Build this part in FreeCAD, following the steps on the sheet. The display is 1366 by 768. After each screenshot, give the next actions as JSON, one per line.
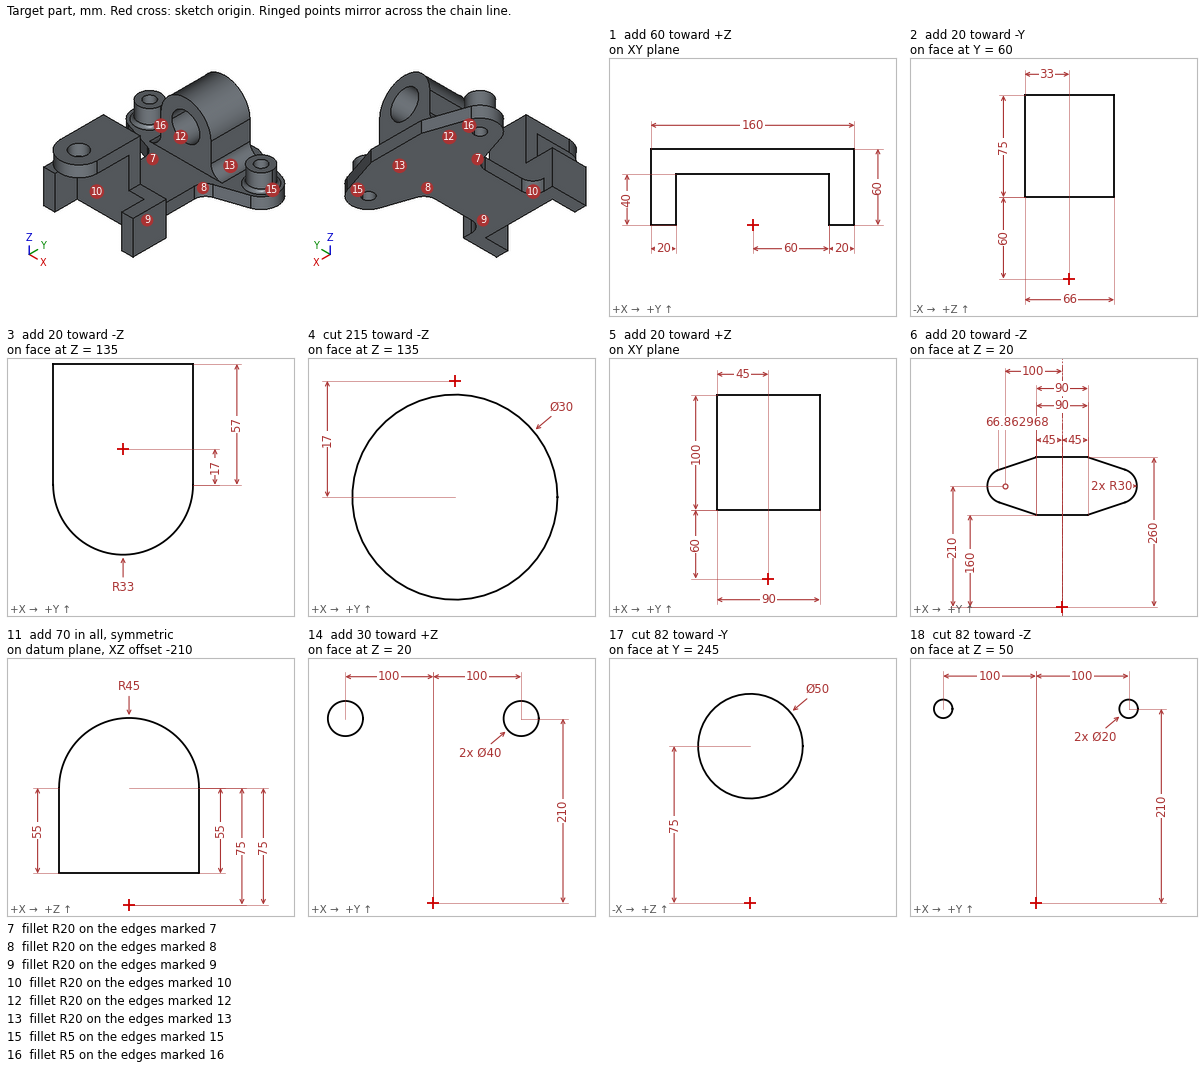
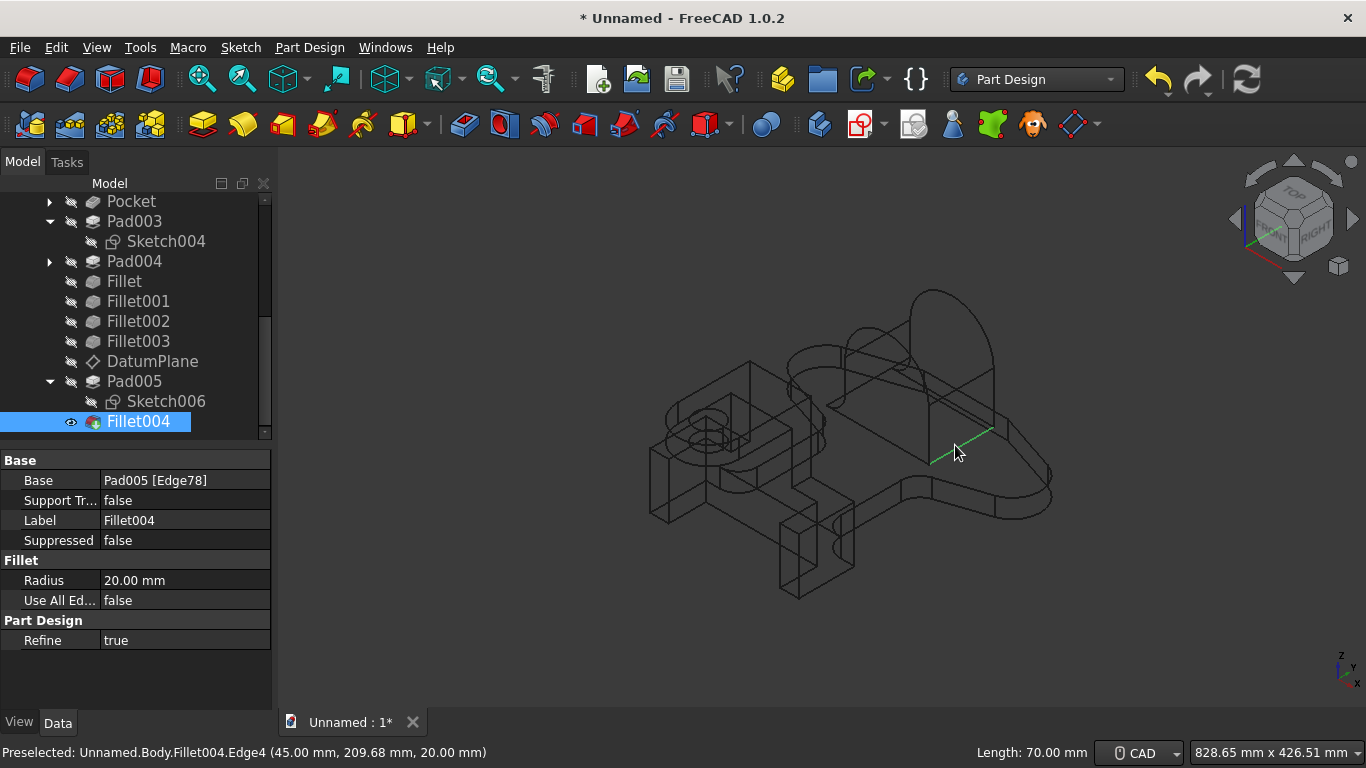
{"action": "key", "text": "v 1"}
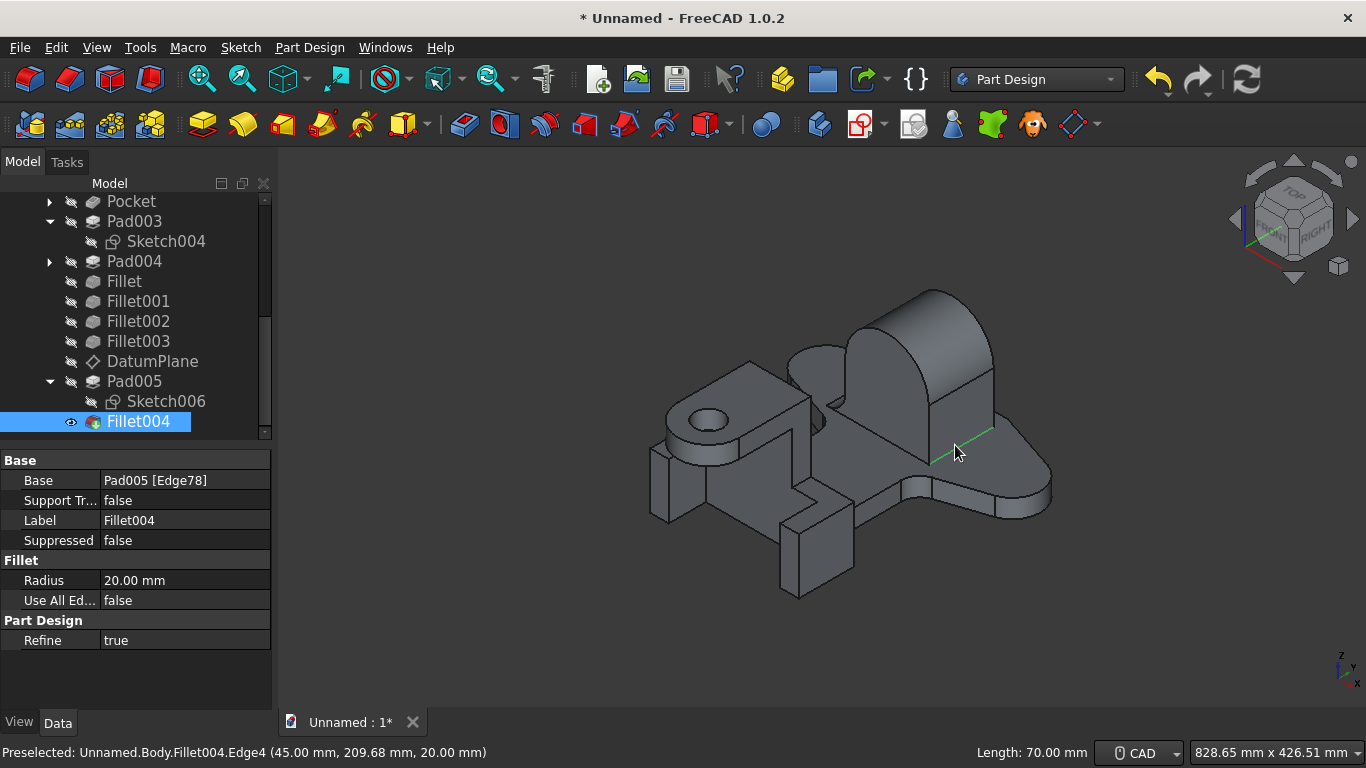
{"action": "left_click", "coordinate": [30, 80]}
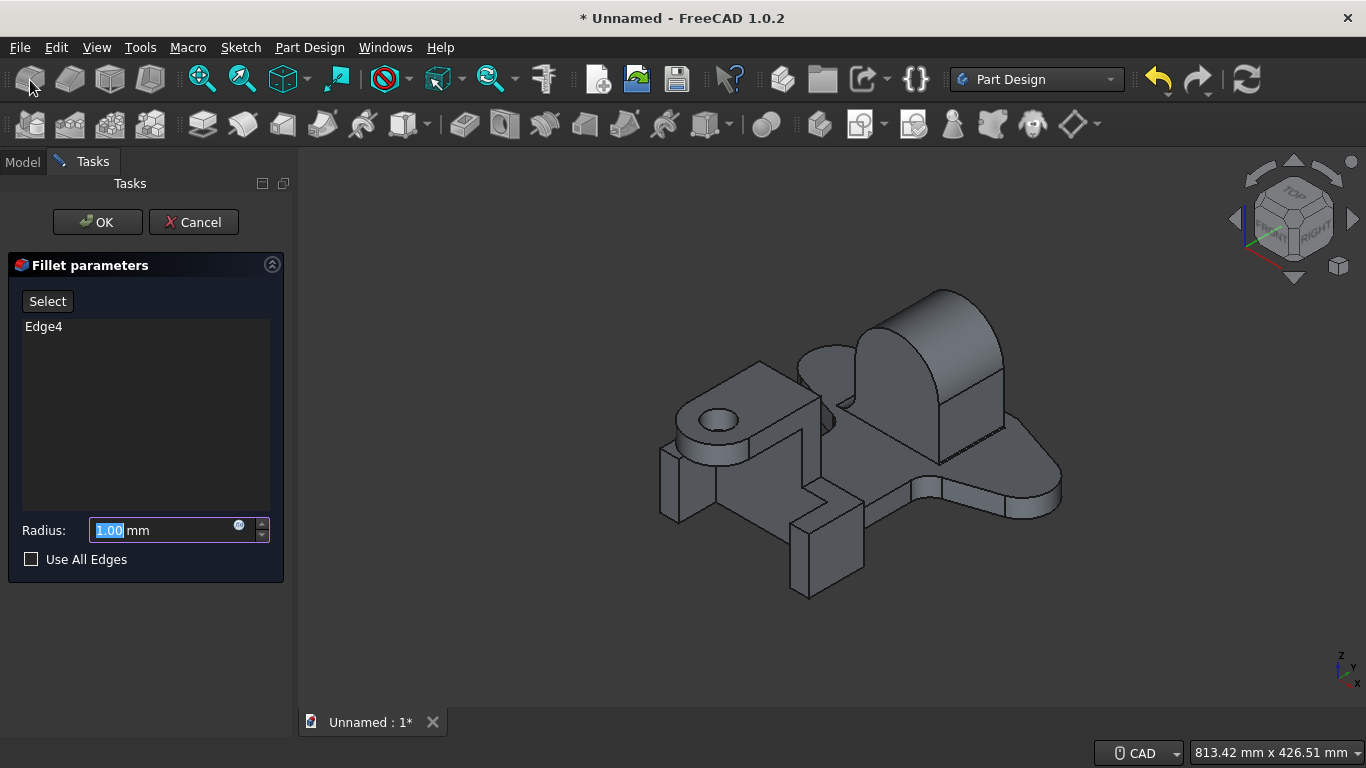
{"action": "type", "text": "20"}
{"action": "key", "text": "Tab"}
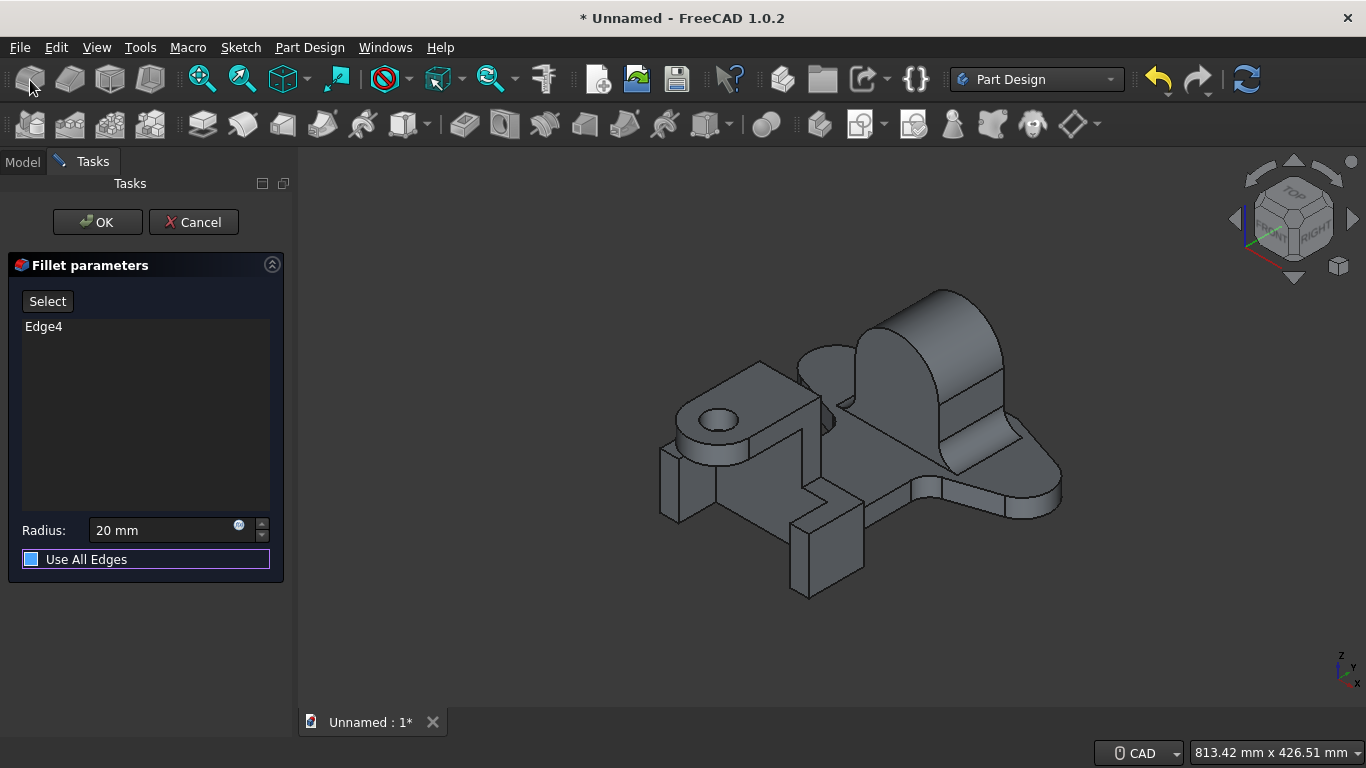
{"action": "left_click", "coordinate": [98, 222]}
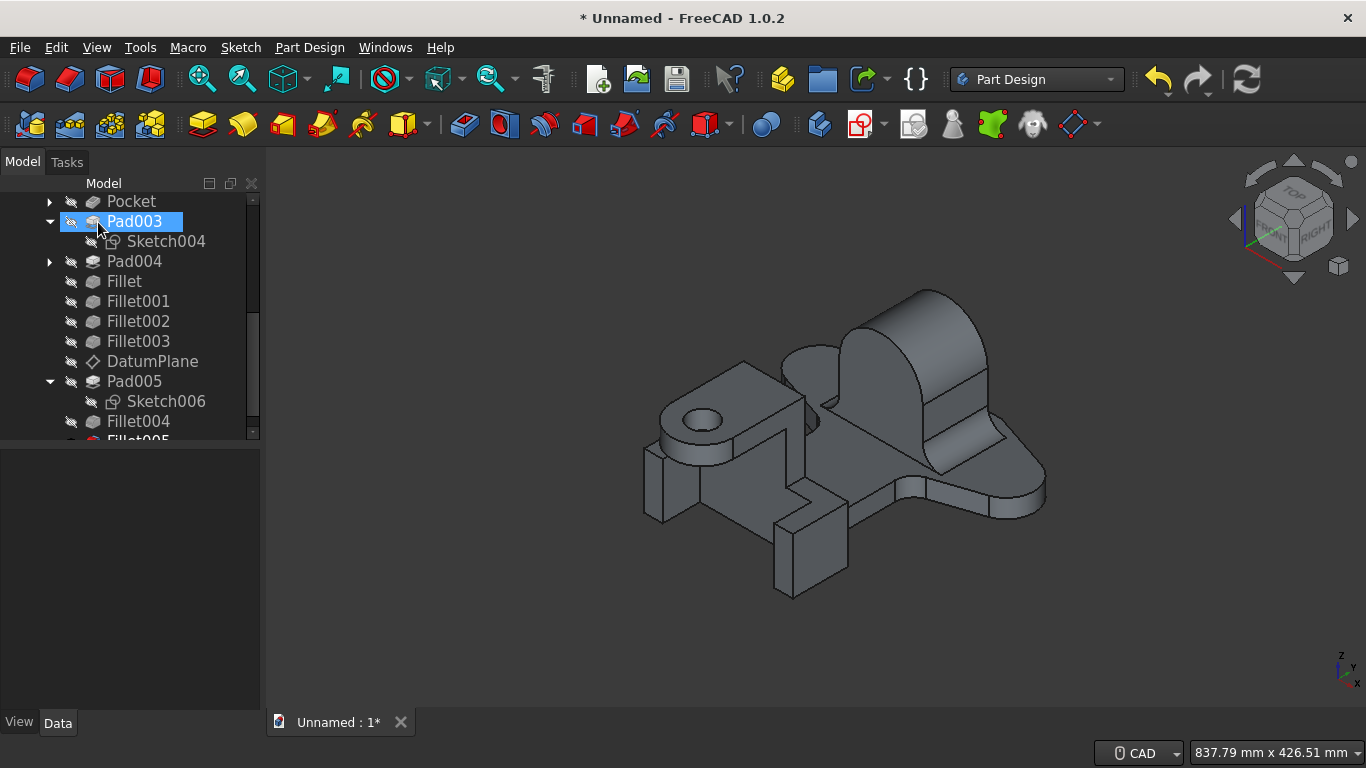
{"action": "left_click", "coordinate": [841, 463]}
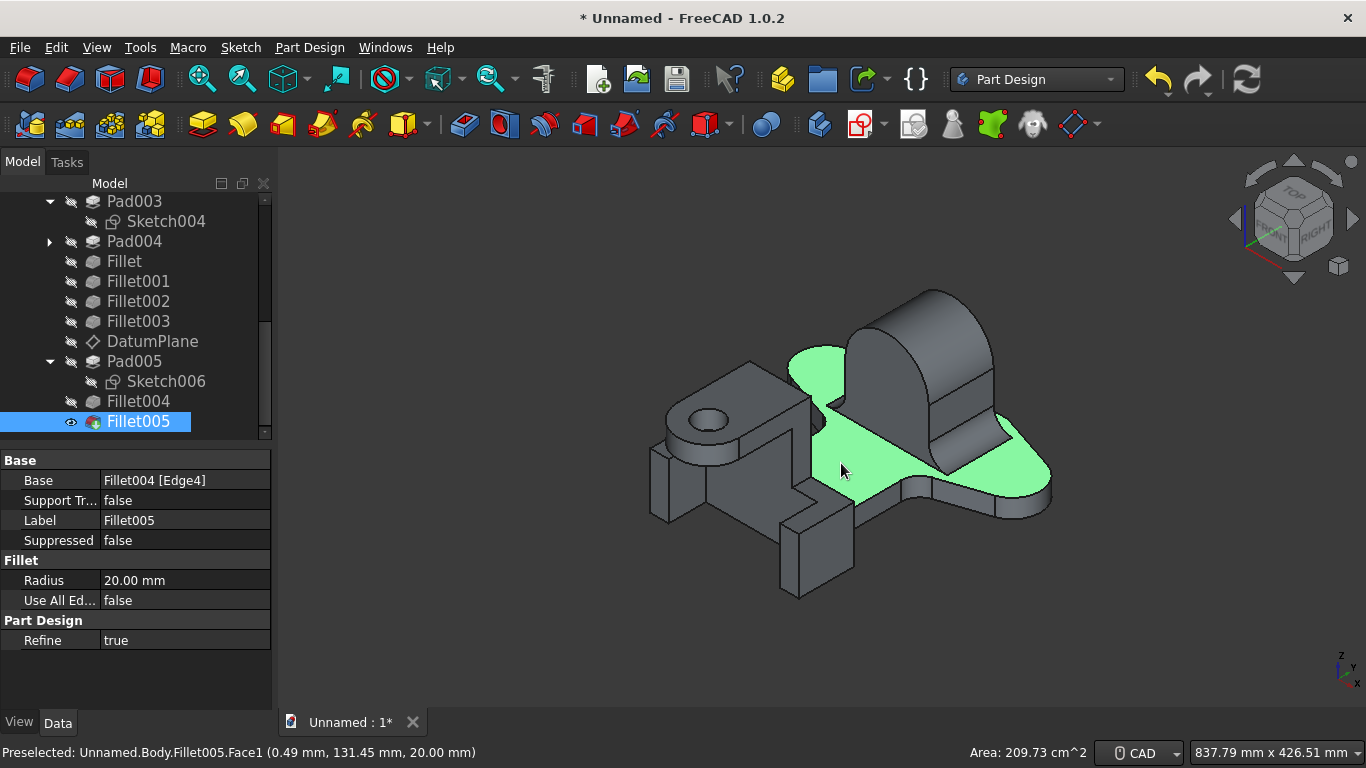
{"action": "left_click", "coordinate": [860, 124]}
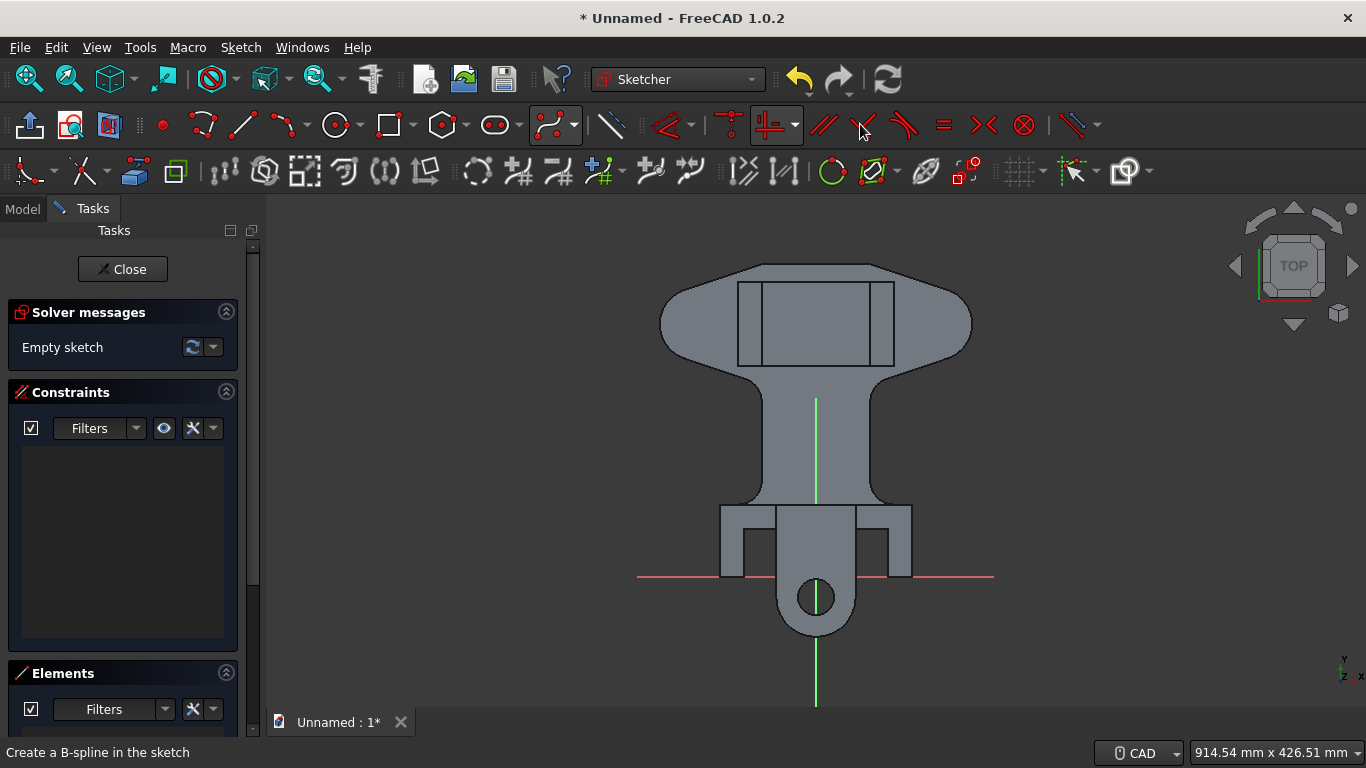
{"action": "key", "text": "g c"}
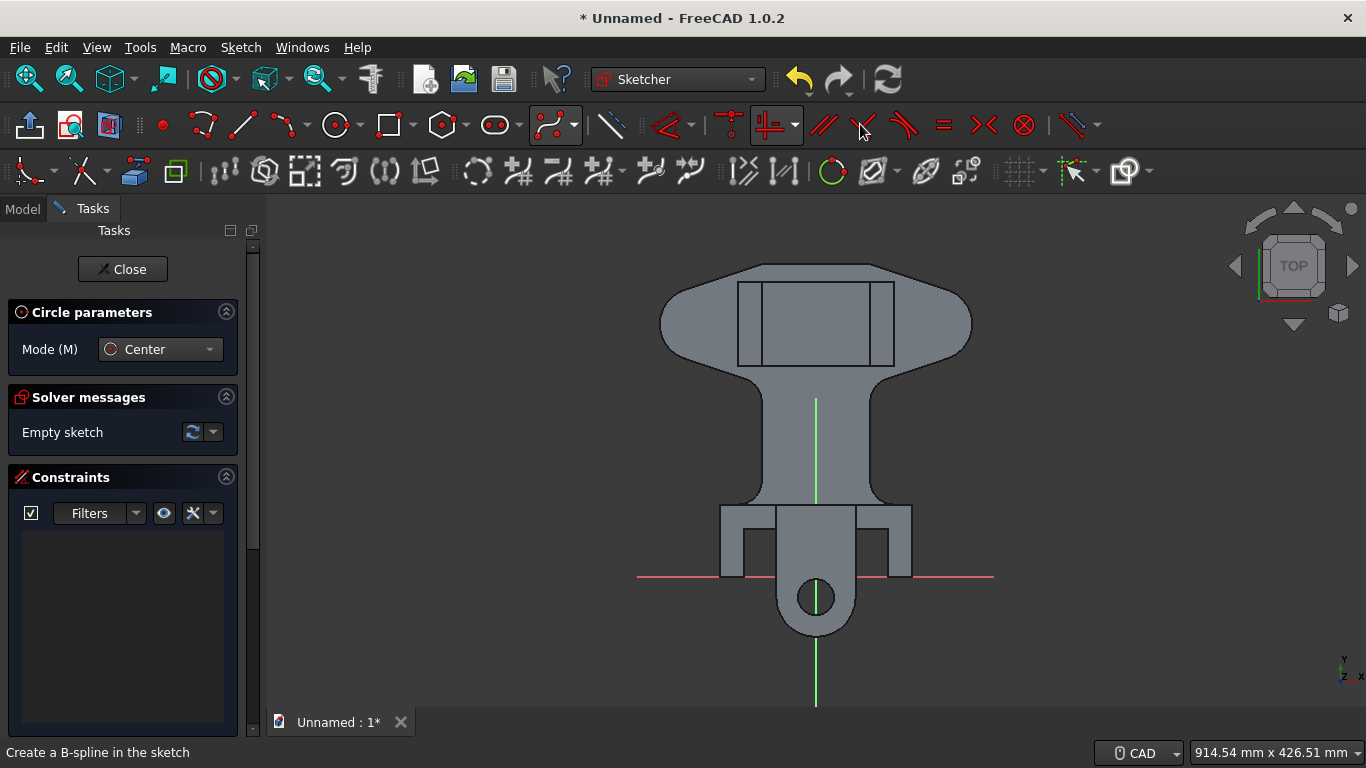
{"action": "left_click", "coordinate": [936, 324]}
{"action": "left_click", "coordinate": [953, 307]}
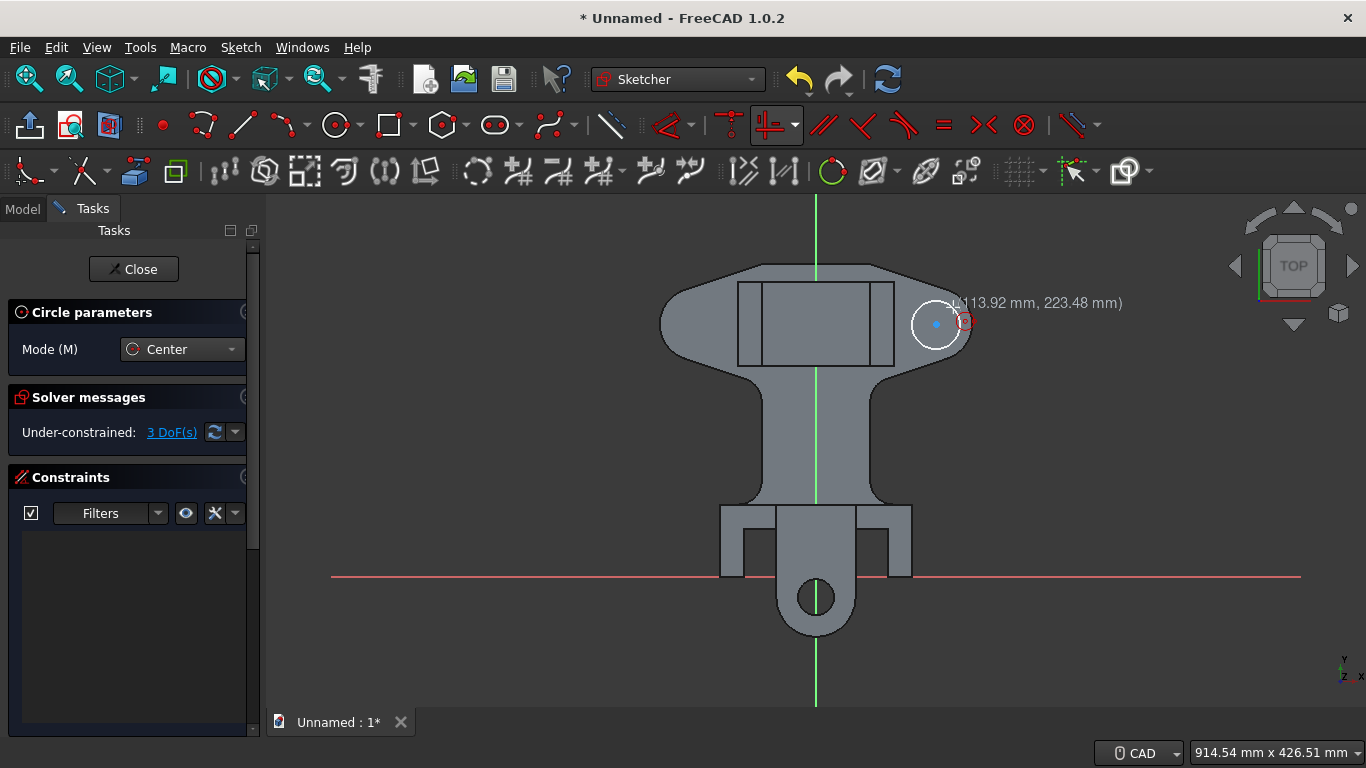
{"action": "left_click", "coordinate": [696, 324]}
{"action": "left_click", "coordinate": [713, 307]}
{"action": "key", "text": "Escape"}